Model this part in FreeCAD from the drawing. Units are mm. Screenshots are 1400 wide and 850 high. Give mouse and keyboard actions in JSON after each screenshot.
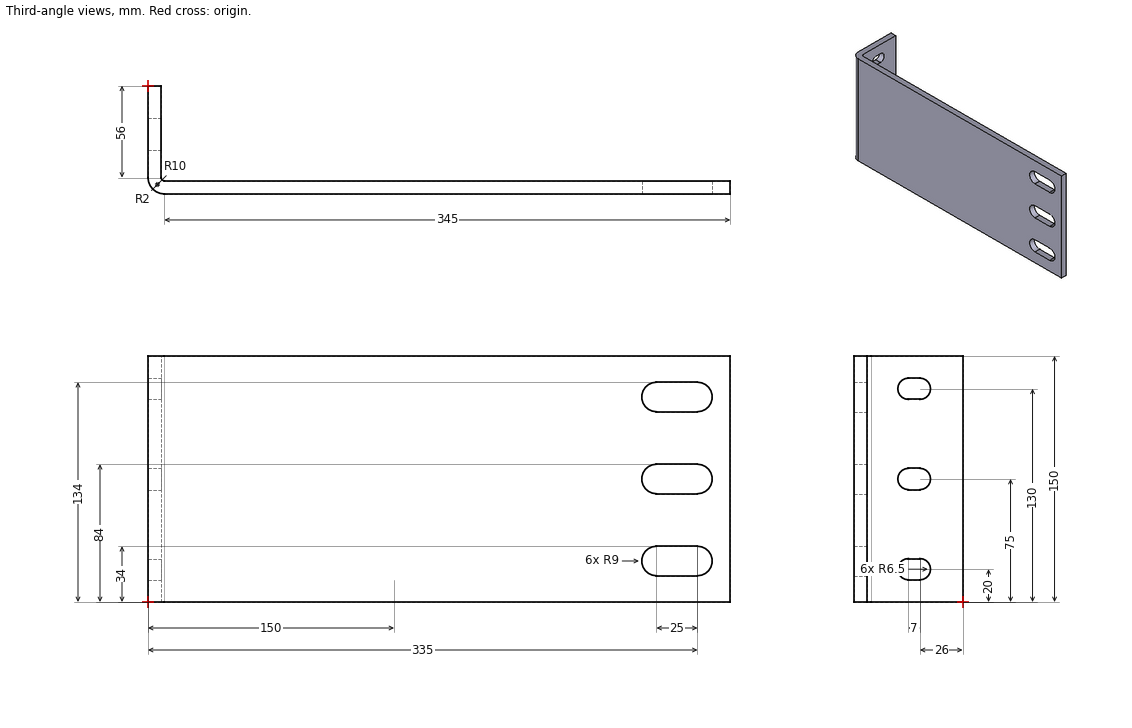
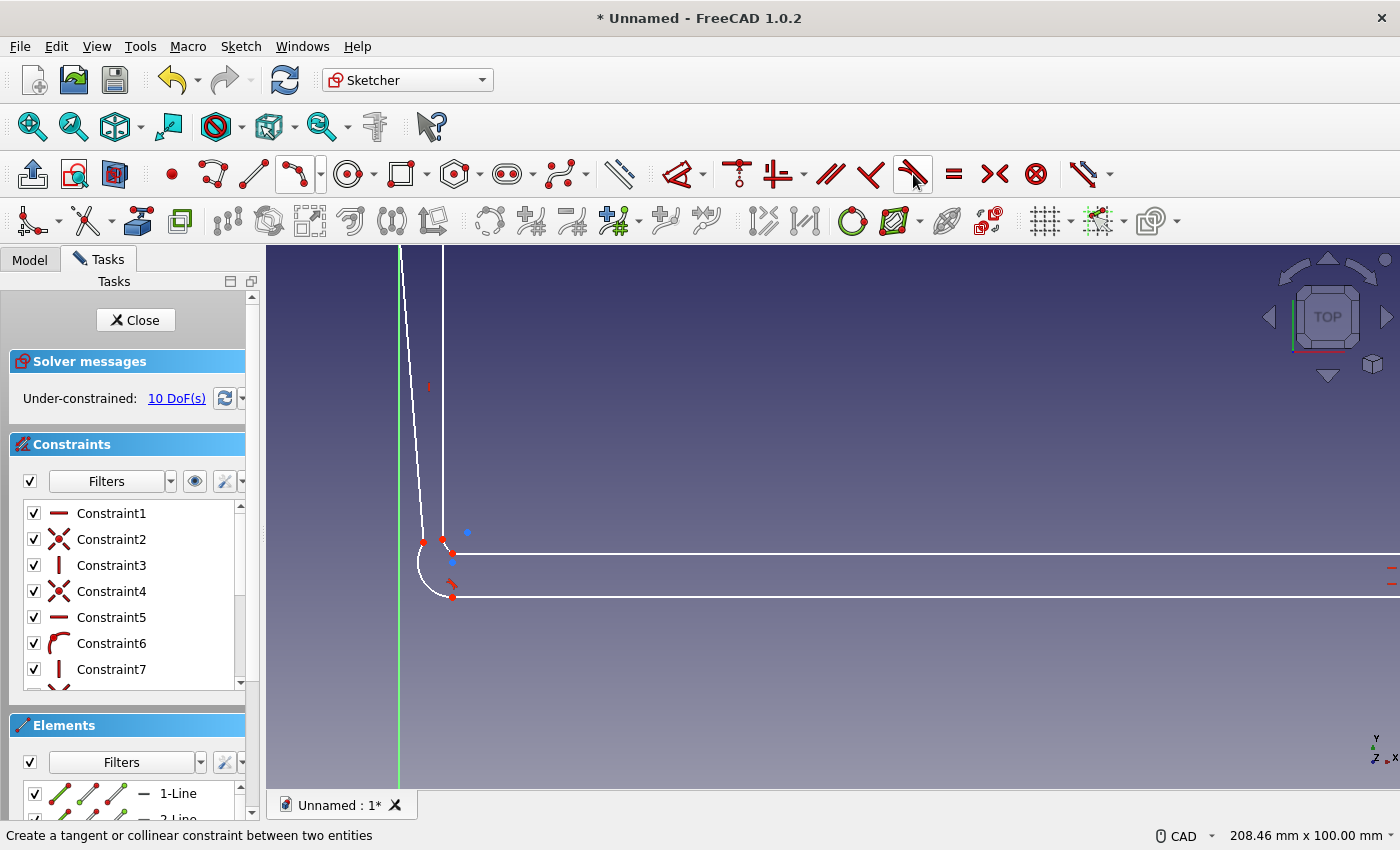
{"action": "left_click", "coordinate": [1016, 554]}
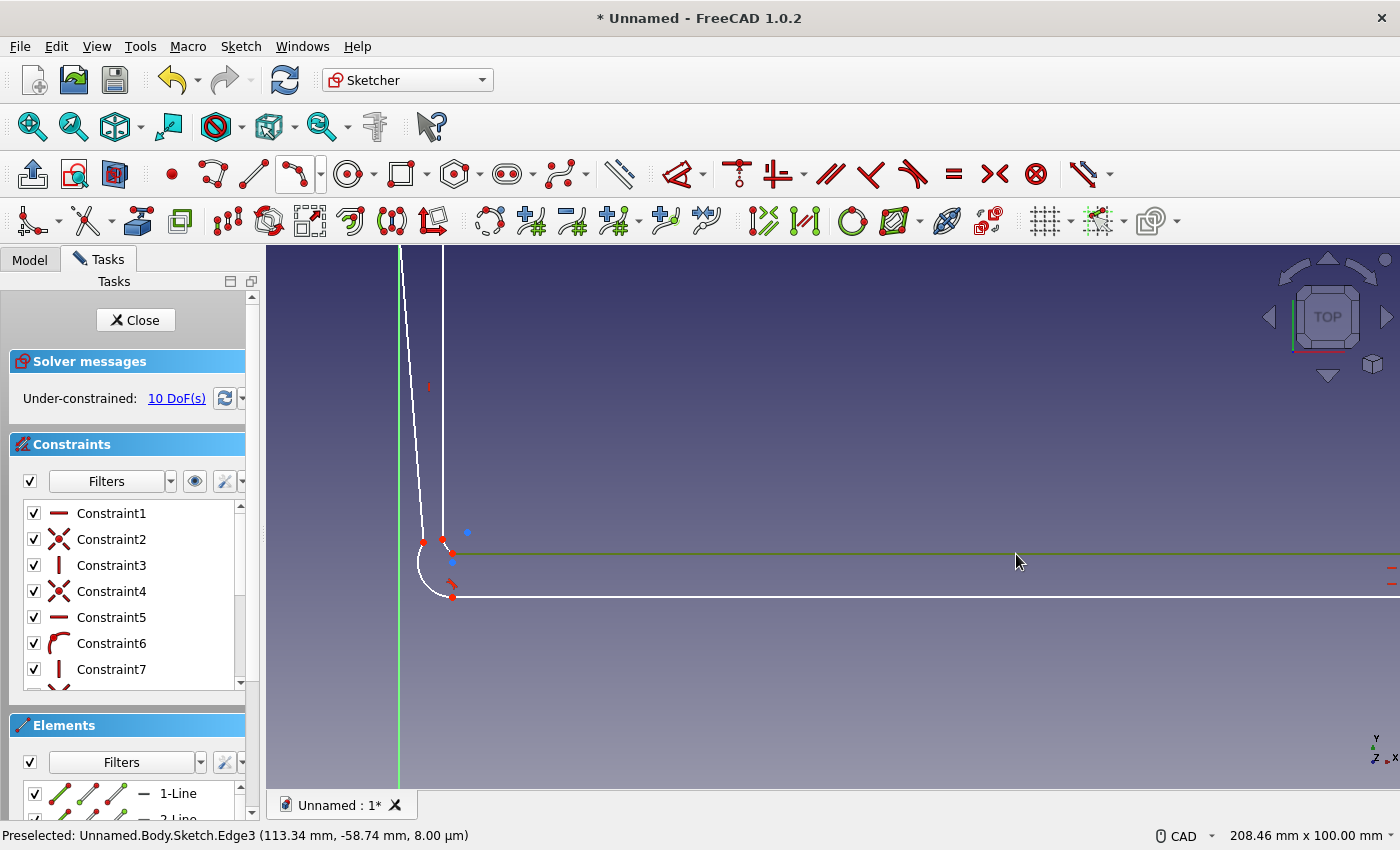
{"action": "scroll", "coordinate": [447, 547], "scroll_direction": "up", "scroll_amount": 3}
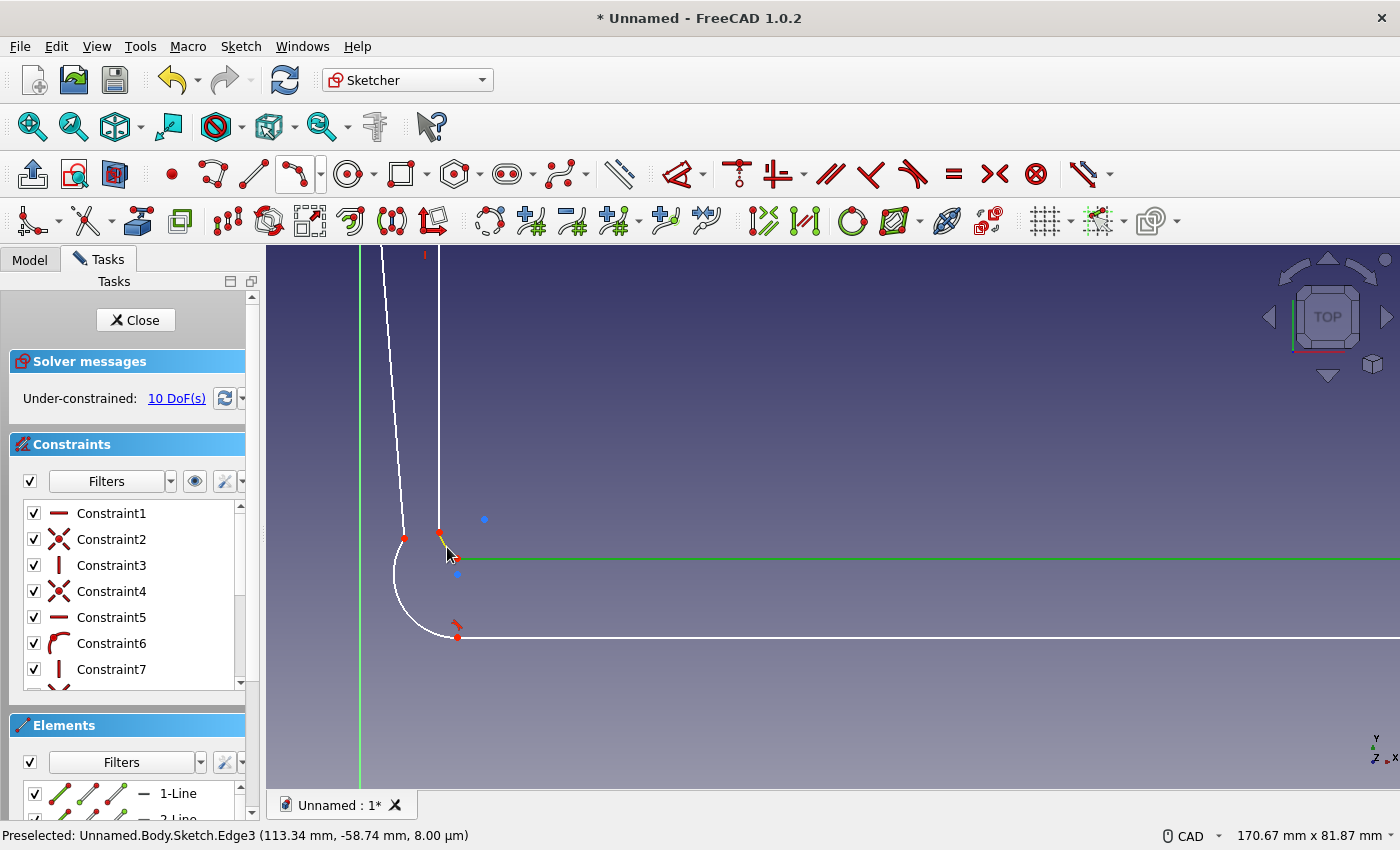
{"action": "left_click", "coordinate": [446, 547]}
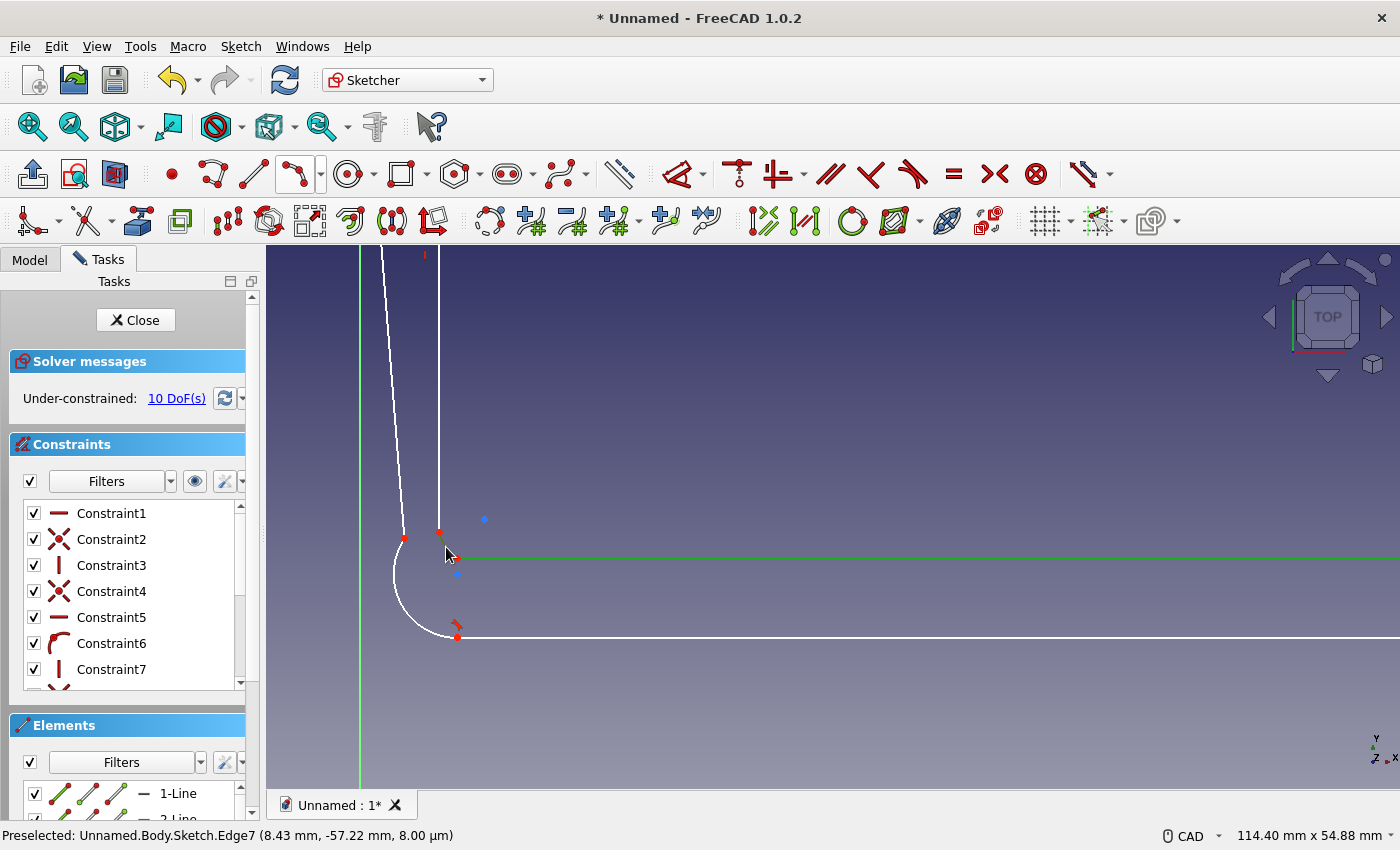
{"action": "left_click", "coordinate": [913, 174]}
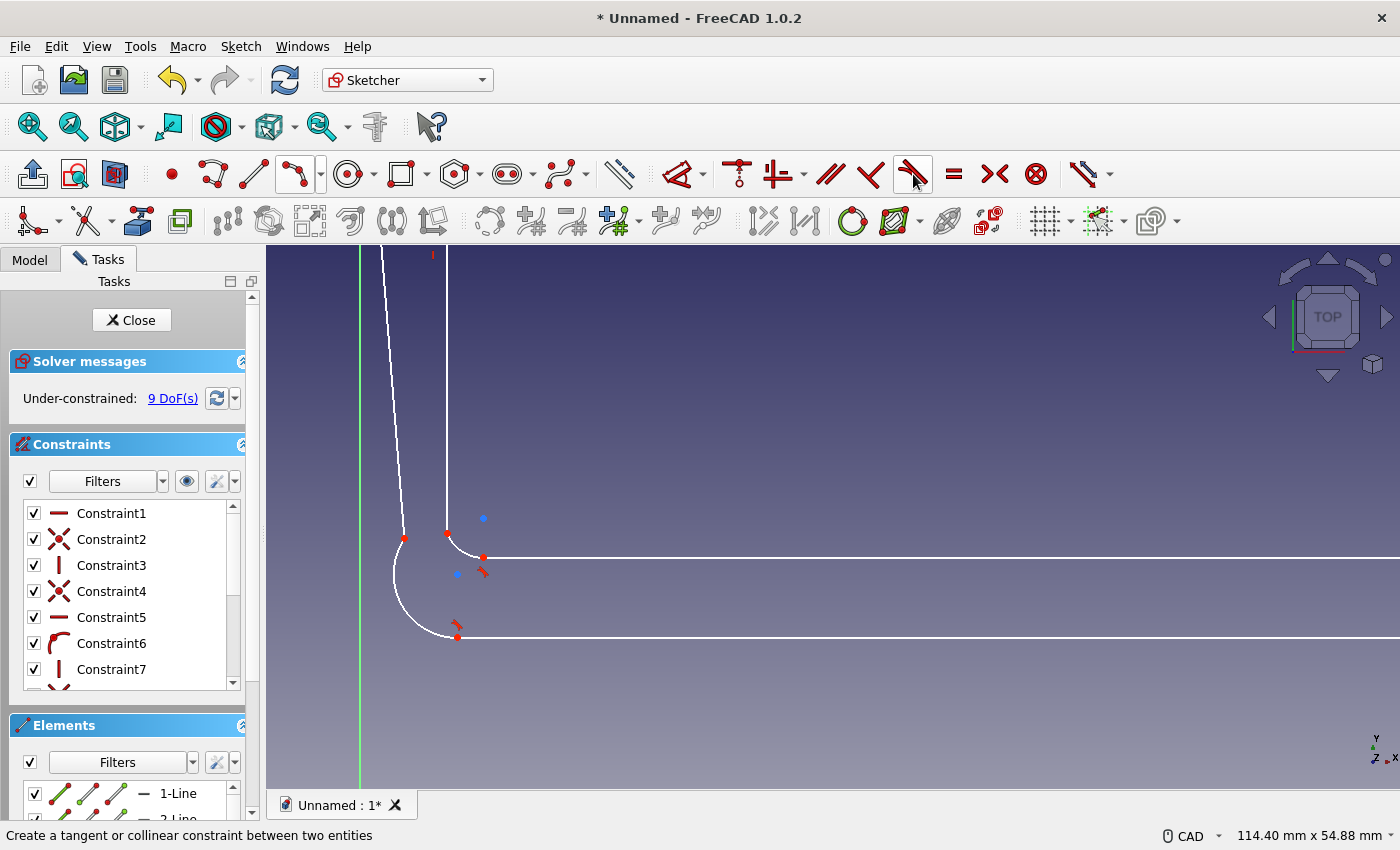
{"action": "scroll", "coordinate": [422, 571], "scroll_direction": "down", "scroll_amount": 8}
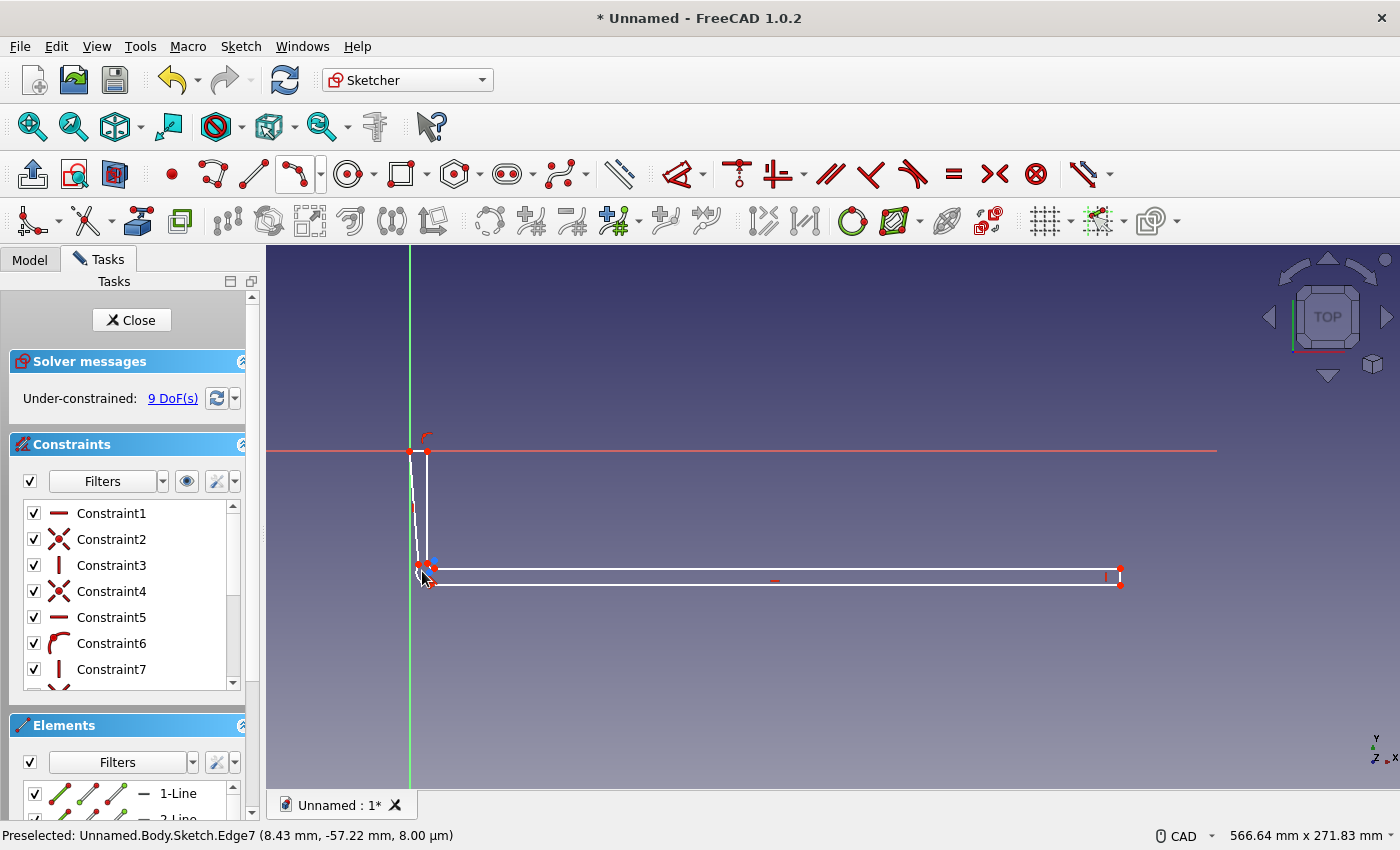
{"action": "left_click", "coordinate": [427, 530]}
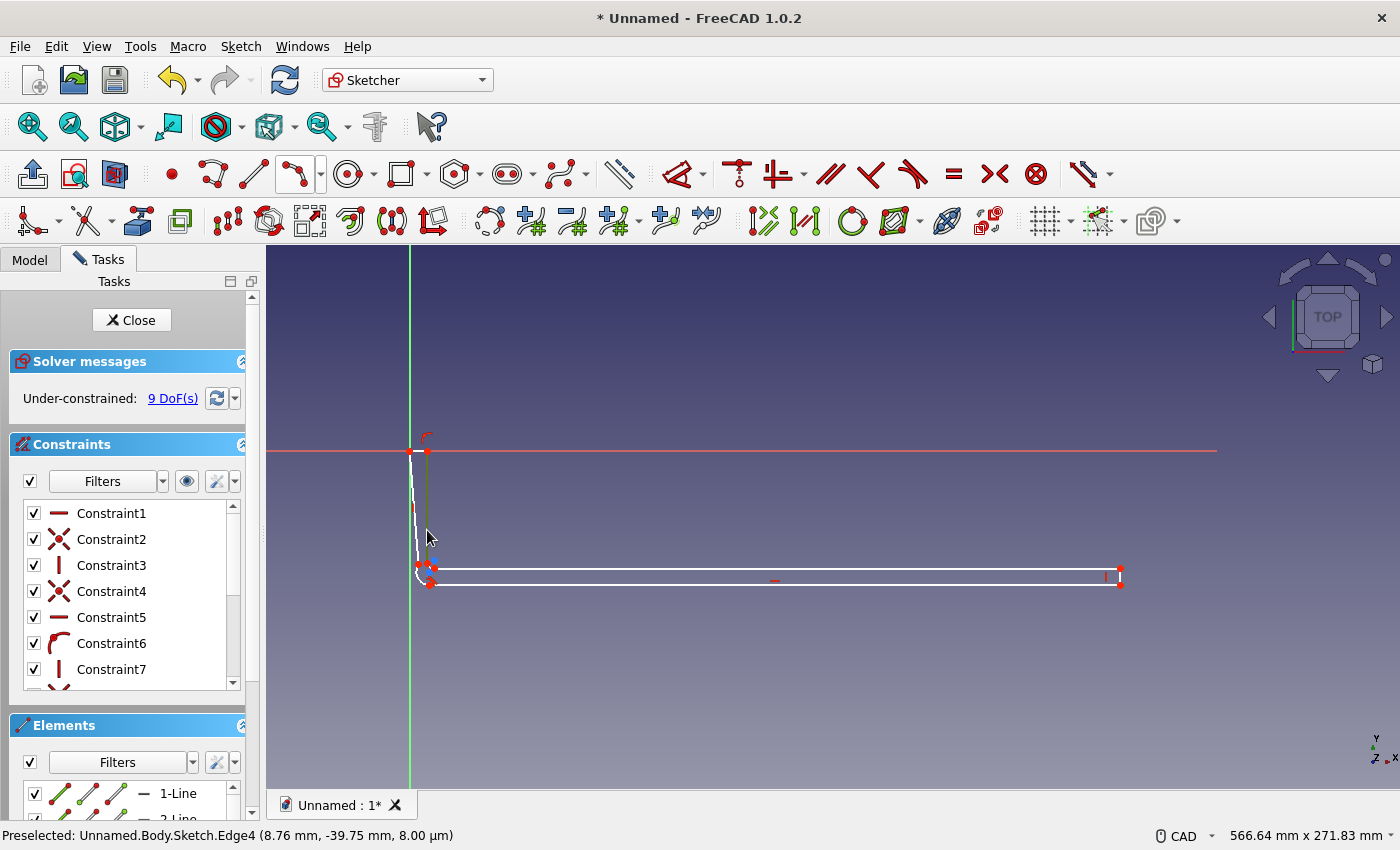
{"action": "scroll", "coordinate": [430, 567], "scroll_direction": "up", "scroll_amount": 6}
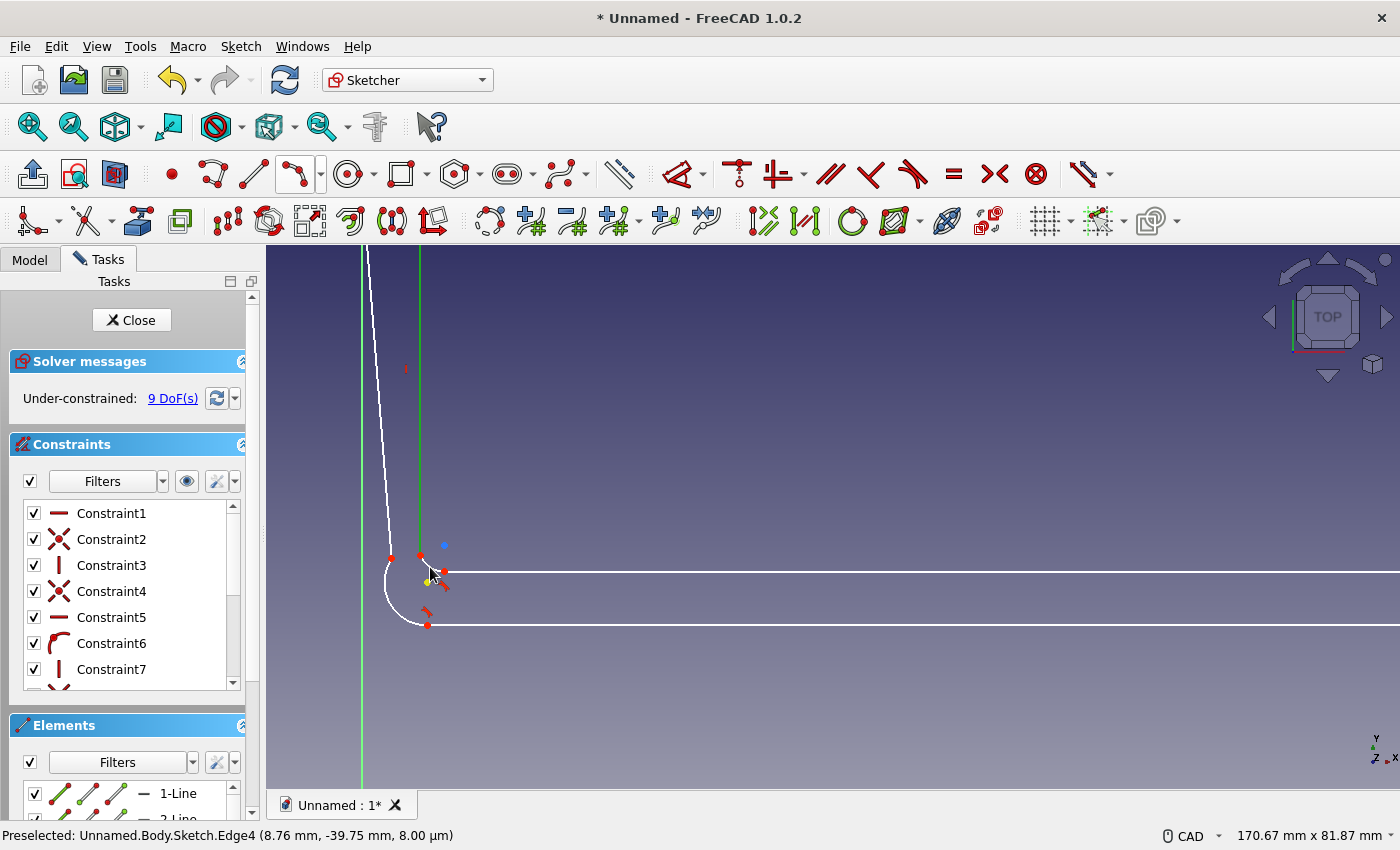
{"action": "left_click", "coordinate": [430, 567]}